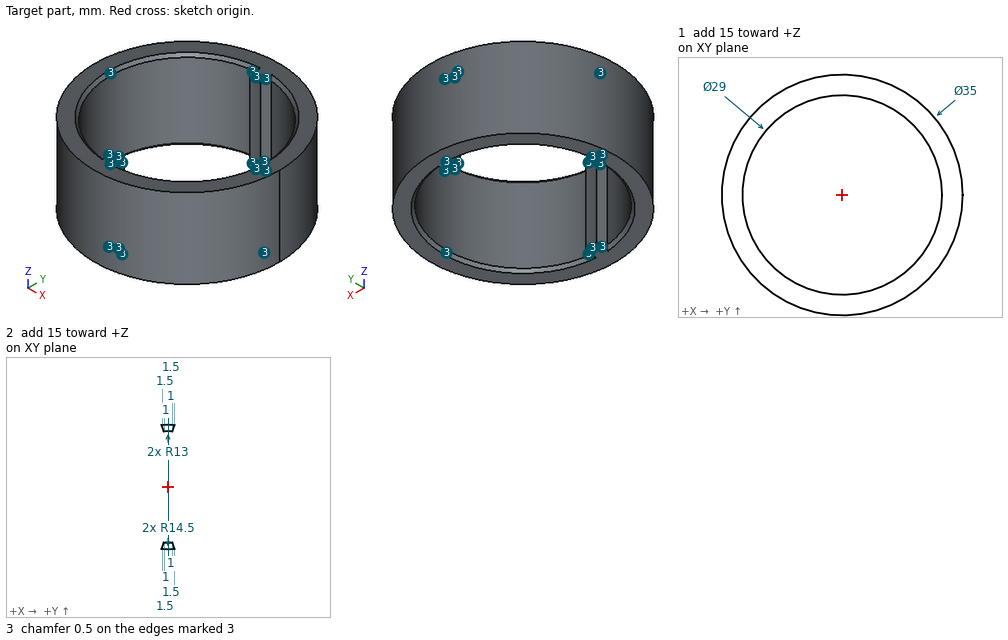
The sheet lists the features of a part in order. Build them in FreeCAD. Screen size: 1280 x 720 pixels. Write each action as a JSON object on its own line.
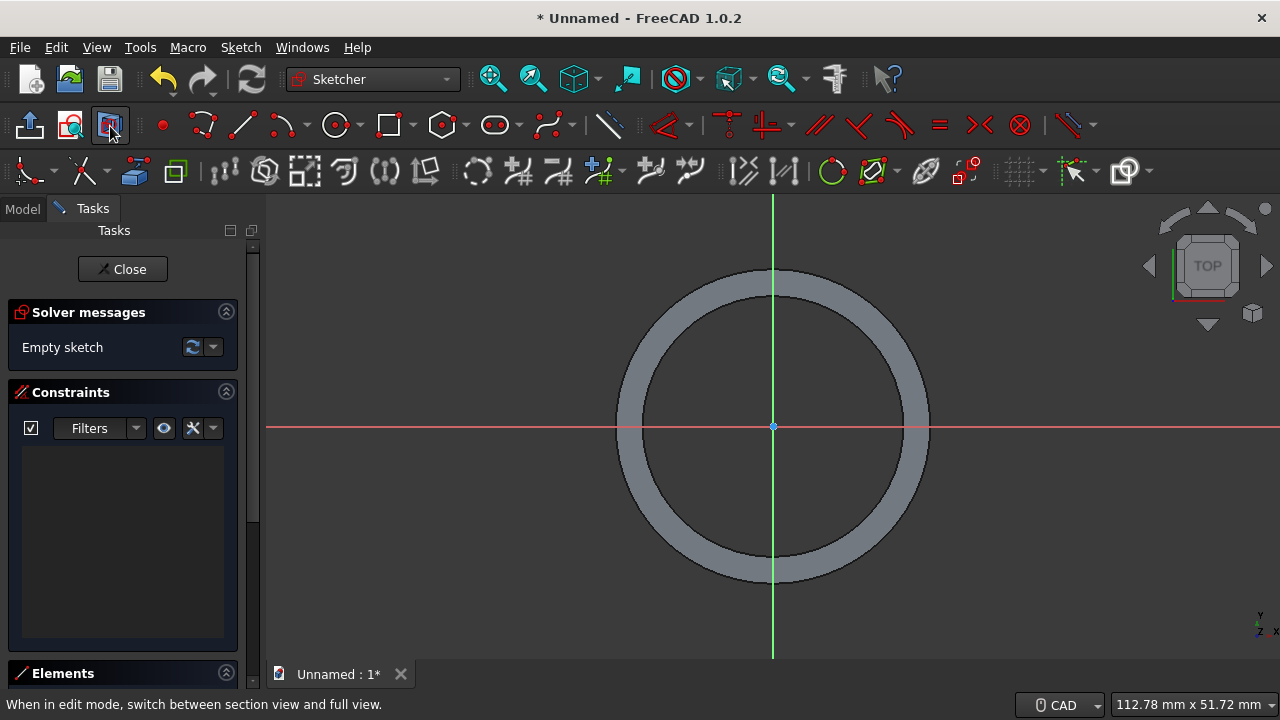
{"action": "left_click", "coordinate": [244, 126]}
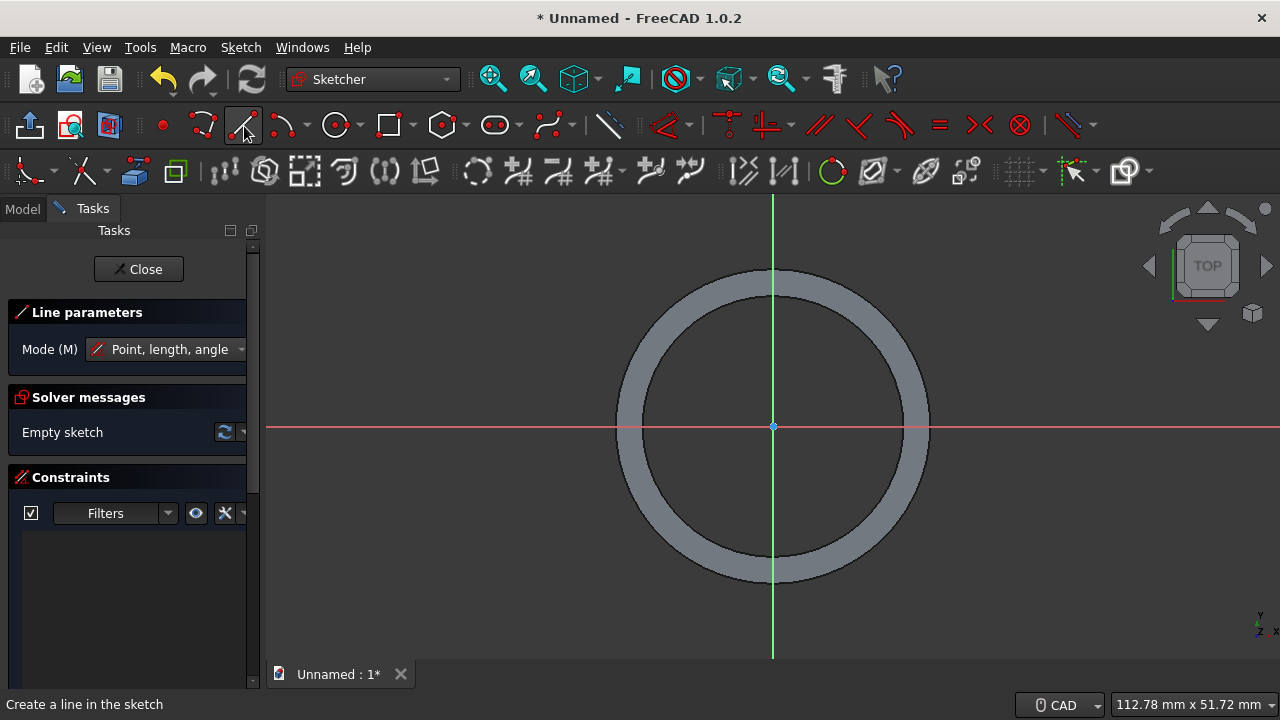
{"action": "left_click", "coordinate": [760, 297]}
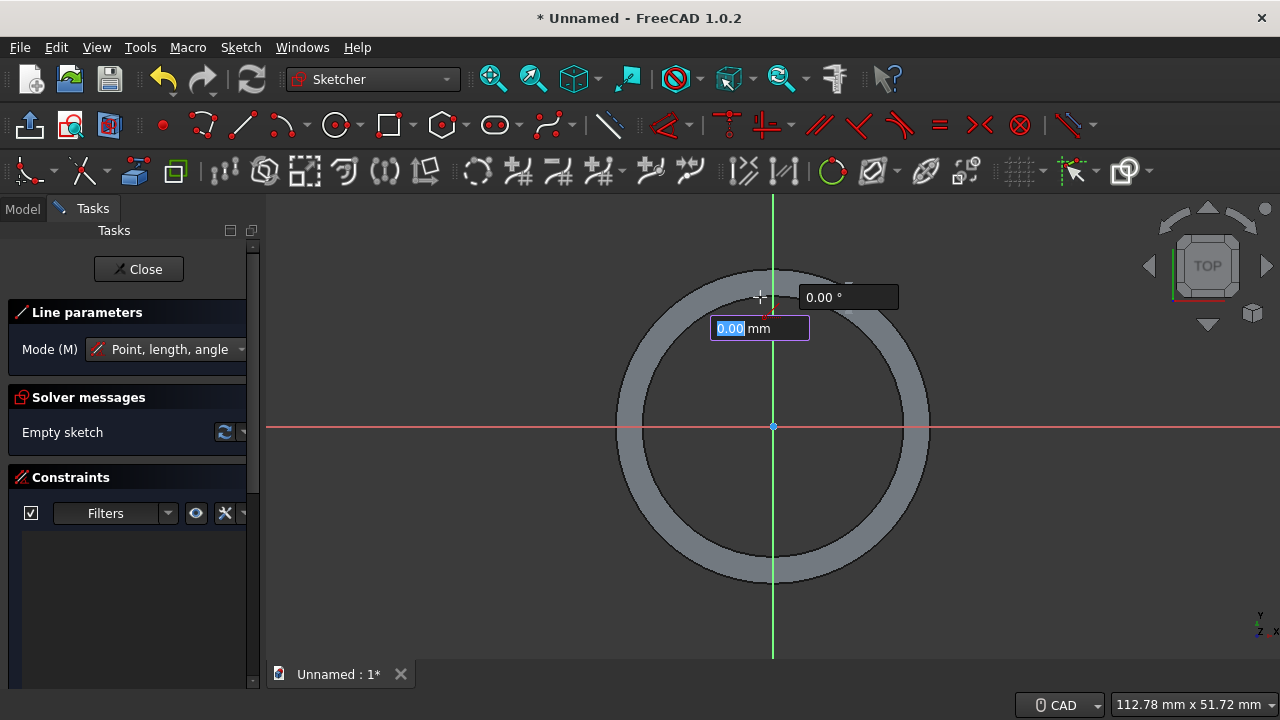
{"action": "scroll", "coordinate": [764, 310], "scroll_direction": "up", "scroll_amount": 3}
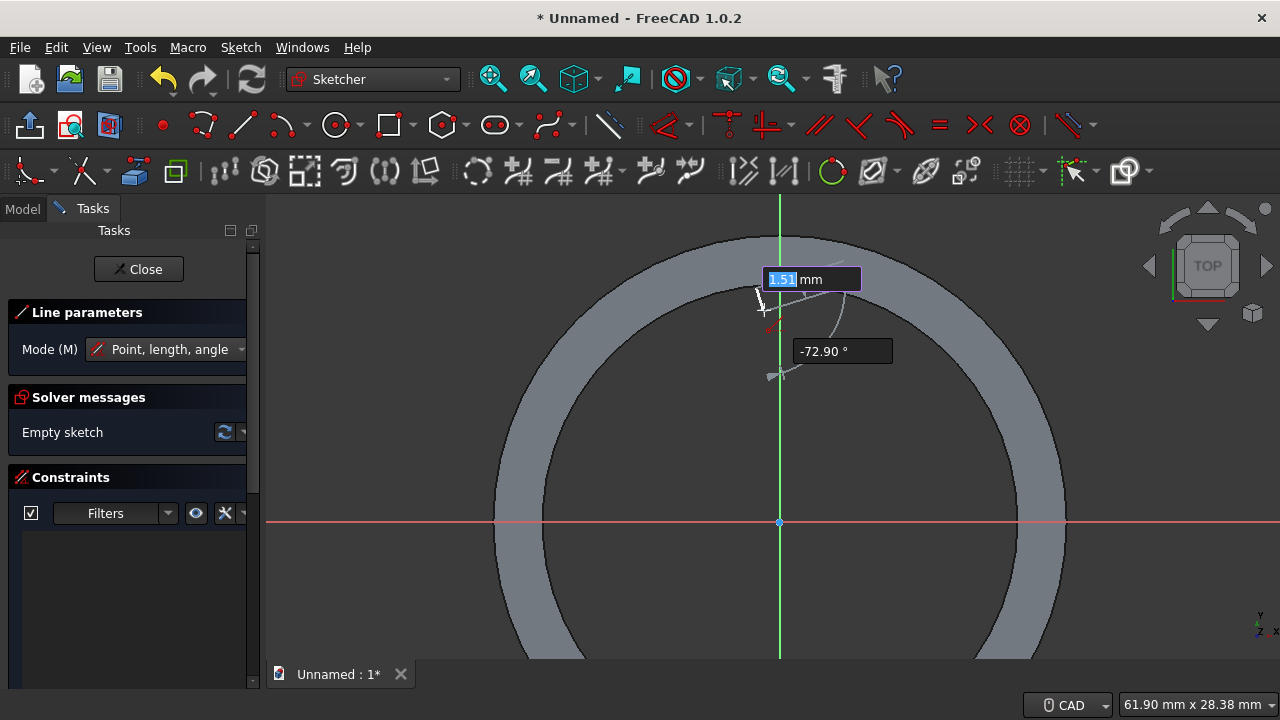
{"action": "left_click", "coordinate": [764, 310]}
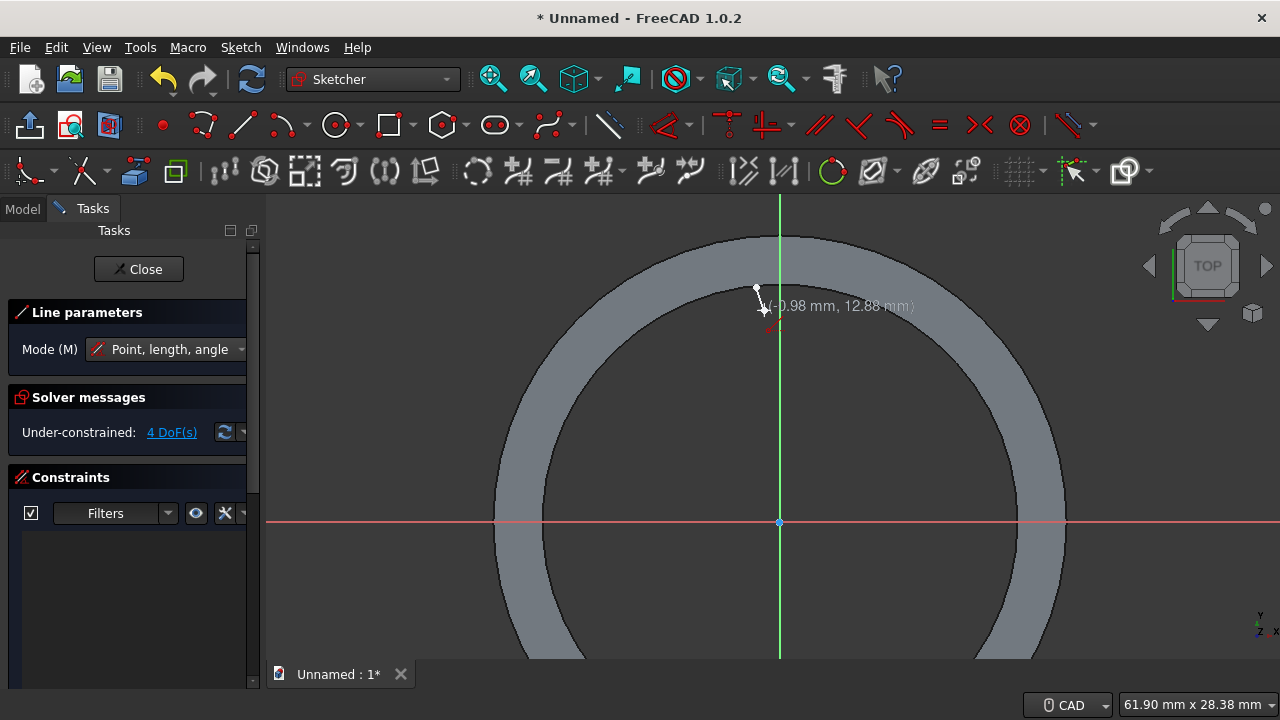
{"action": "left_click", "coordinate": [796, 310]}
{"action": "left_click", "coordinate": [805, 286]}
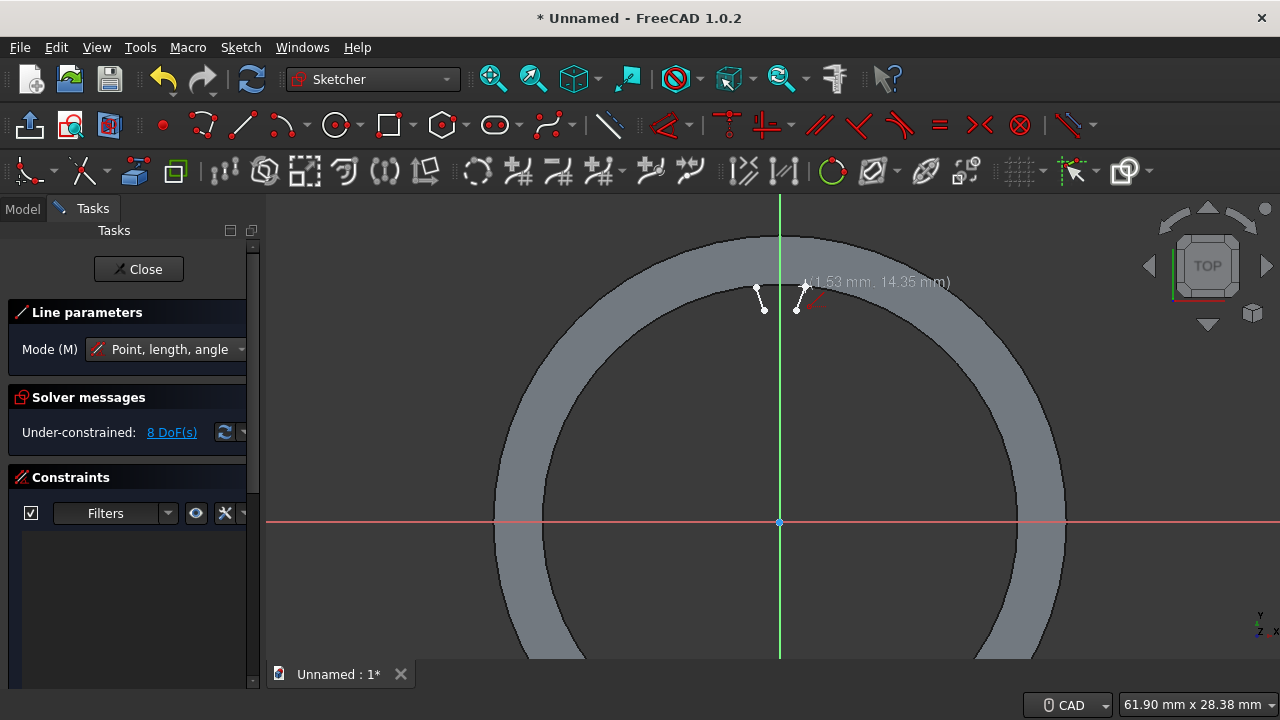
{"action": "left_click", "coordinate": [310, 126]}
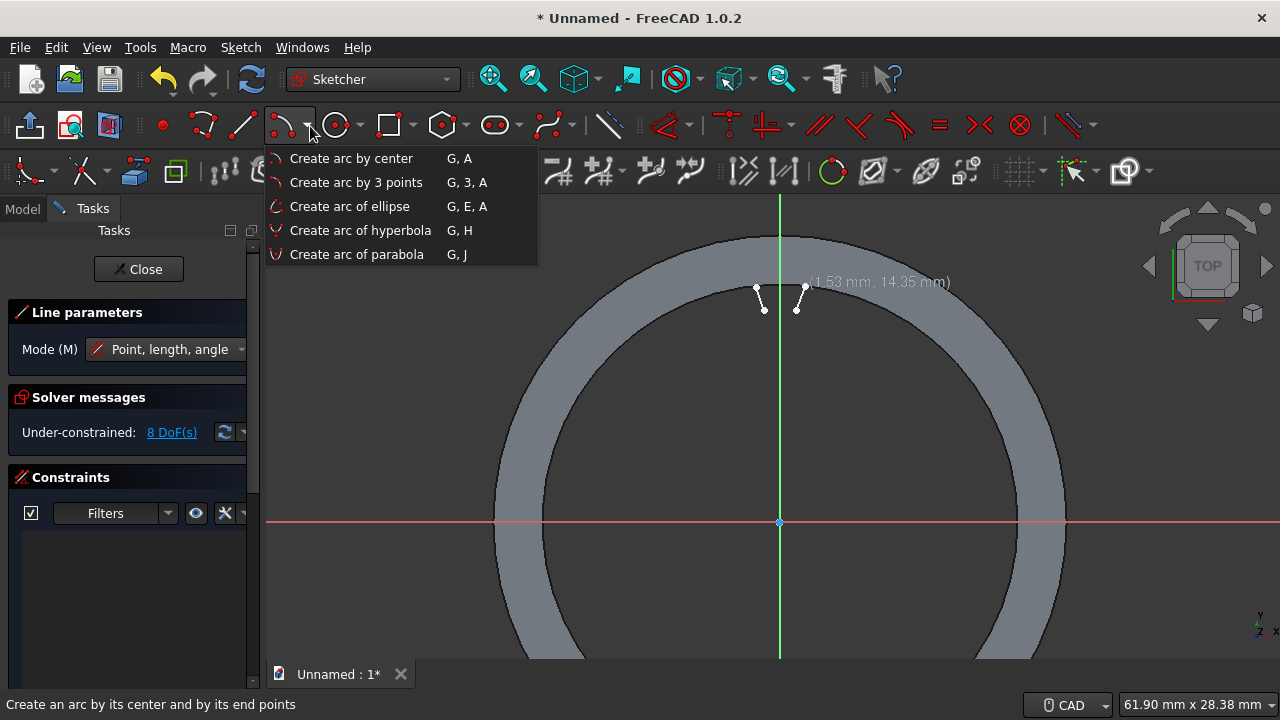
{"action": "left_click", "coordinate": [402, 182]}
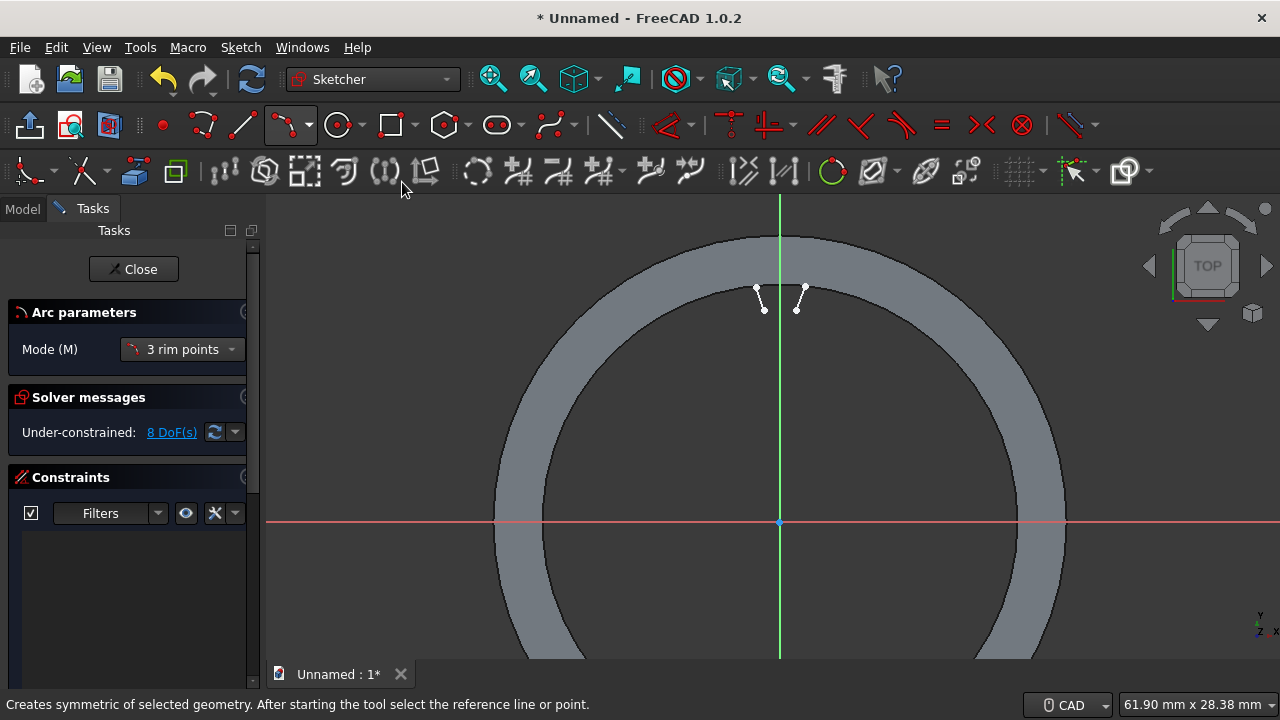
{"action": "scroll", "coordinate": [764, 310], "scroll_direction": "up", "scroll_amount": 2}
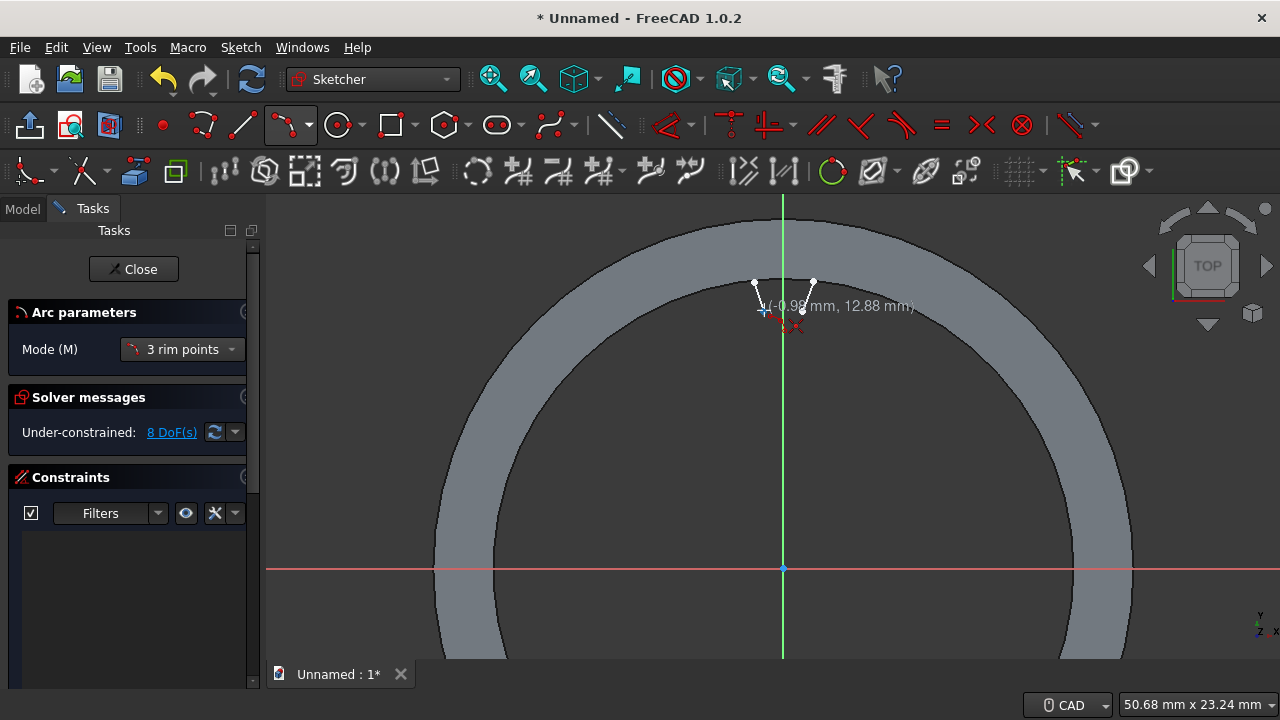
{"action": "left_click", "coordinate": [764, 311]}
{"action": "left_click", "coordinate": [811, 311]}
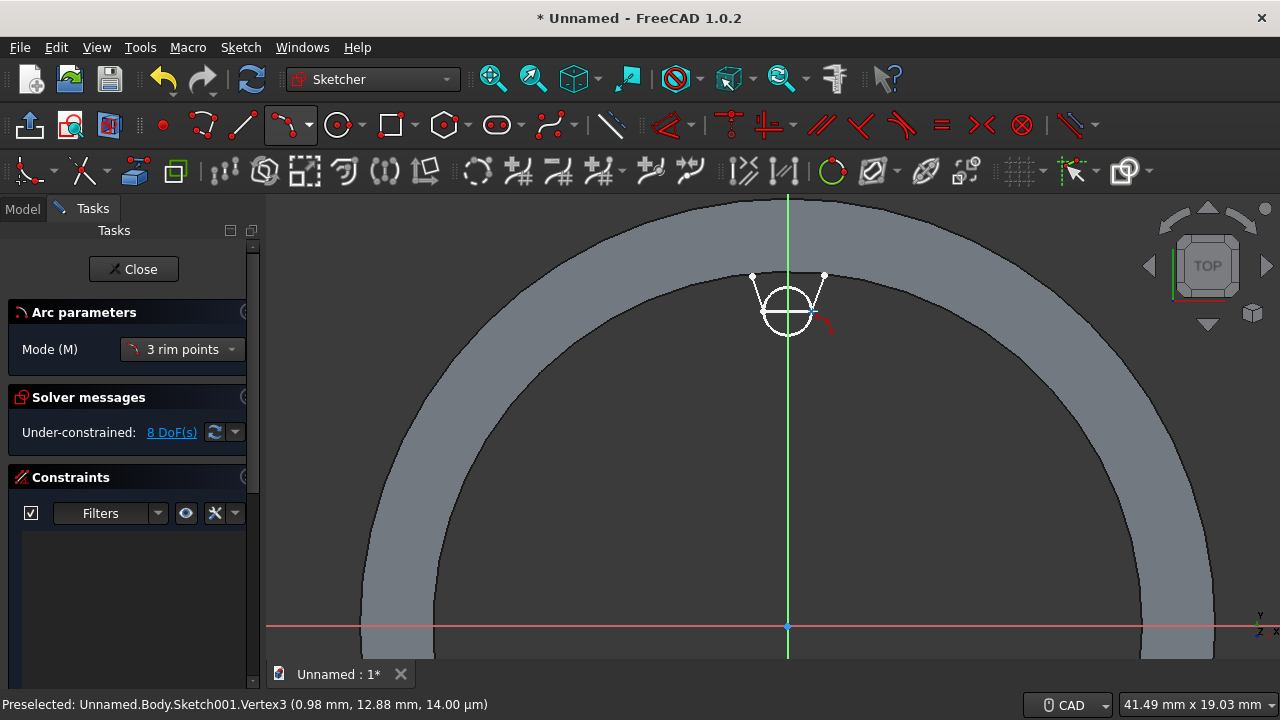
{"action": "scroll", "coordinate": [793, 309], "scroll_direction": "up", "scroll_amount": 15}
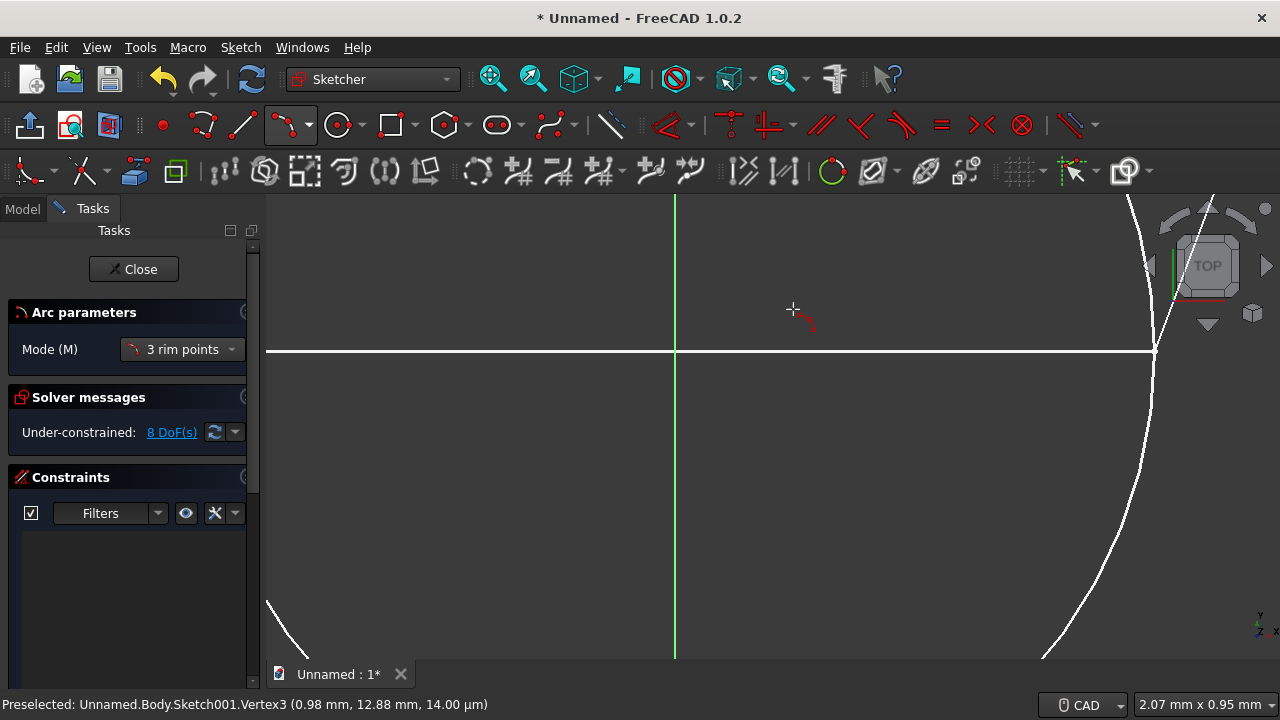
{"action": "left_click", "coordinate": [773, 296]}